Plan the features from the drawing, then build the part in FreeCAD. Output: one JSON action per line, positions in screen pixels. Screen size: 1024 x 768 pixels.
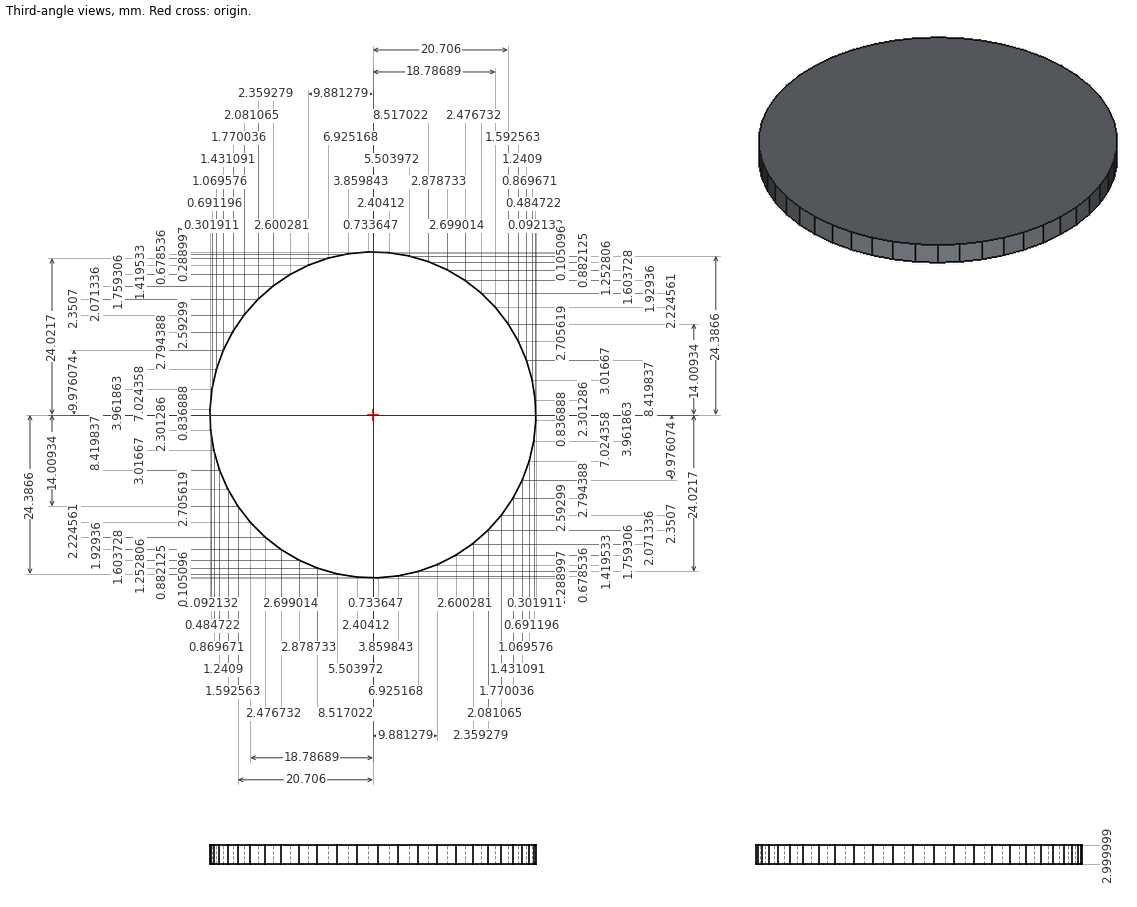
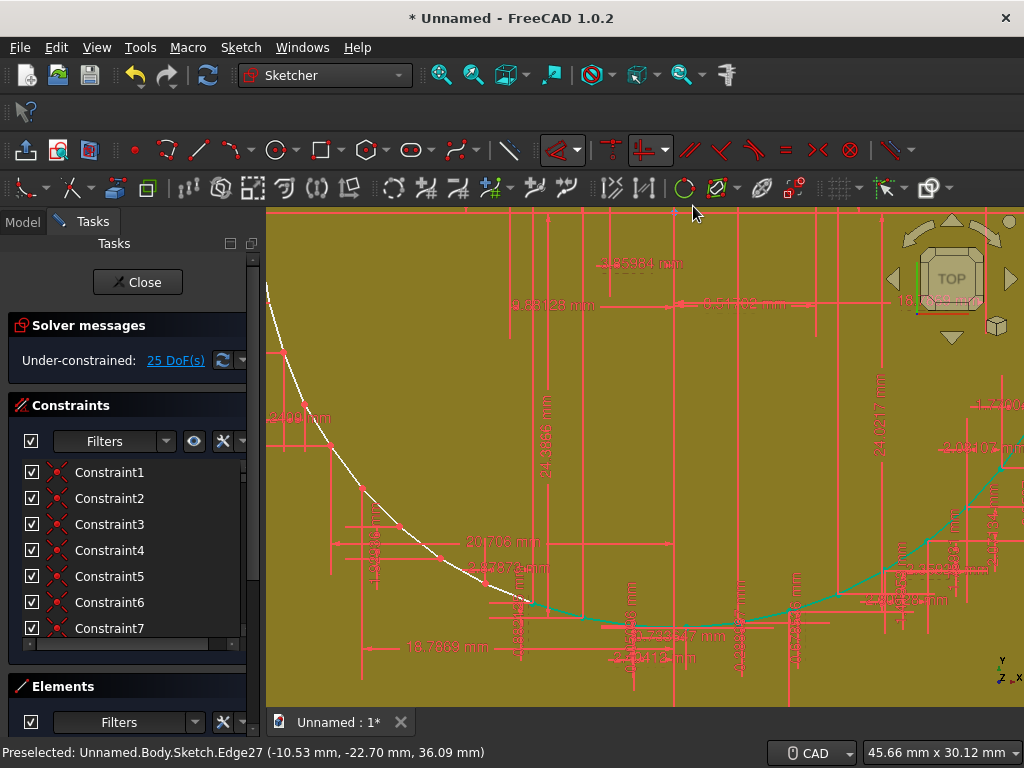
{"action": "scroll", "coordinate": [519, 597], "scroll_direction": "up", "scroll_amount": 4}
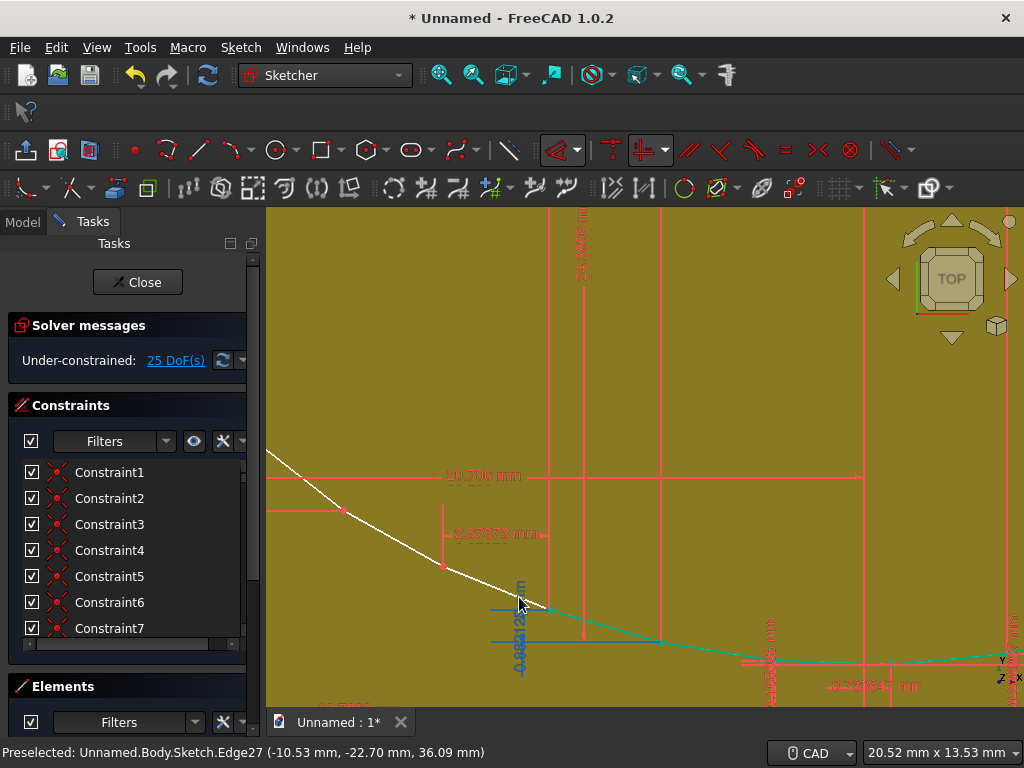
{"action": "left_click", "coordinate": [475, 579]}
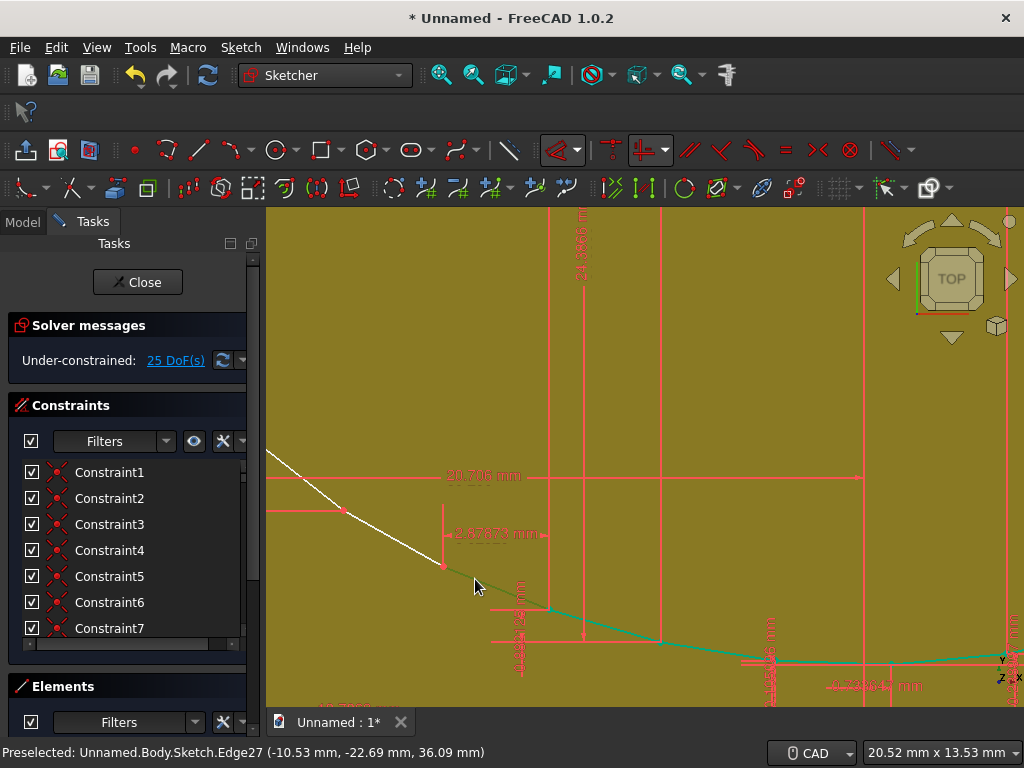
{"action": "left_click", "coordinate": [580, 150]}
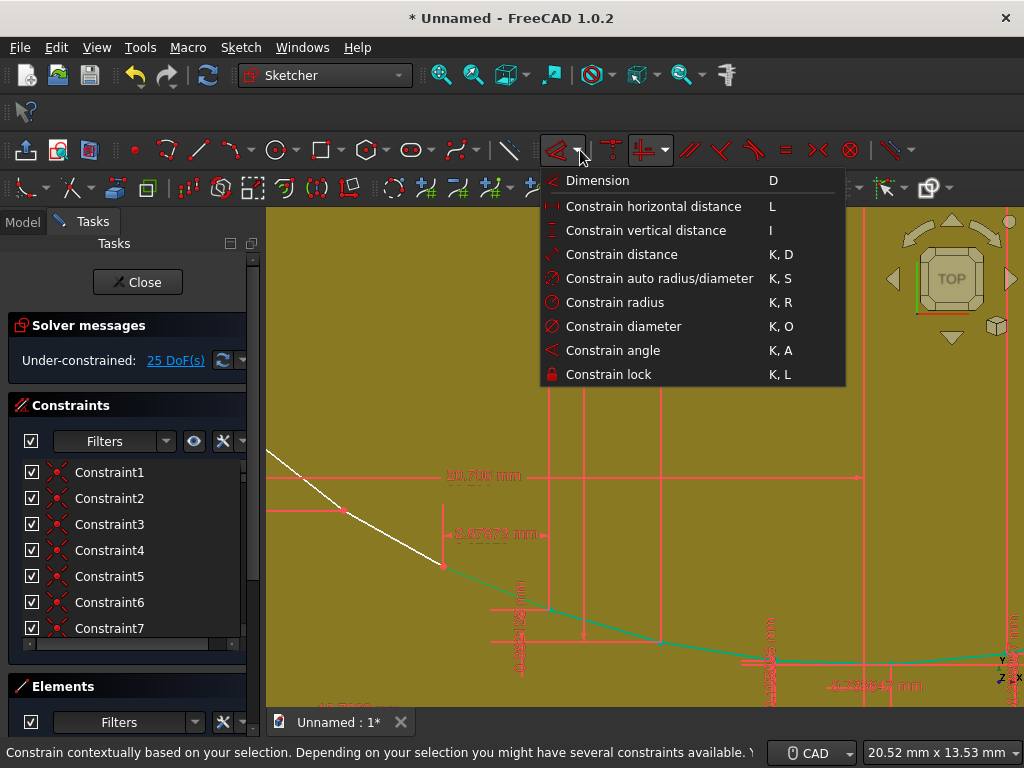
{"action": "left_click", "coordinate": [693, 230]}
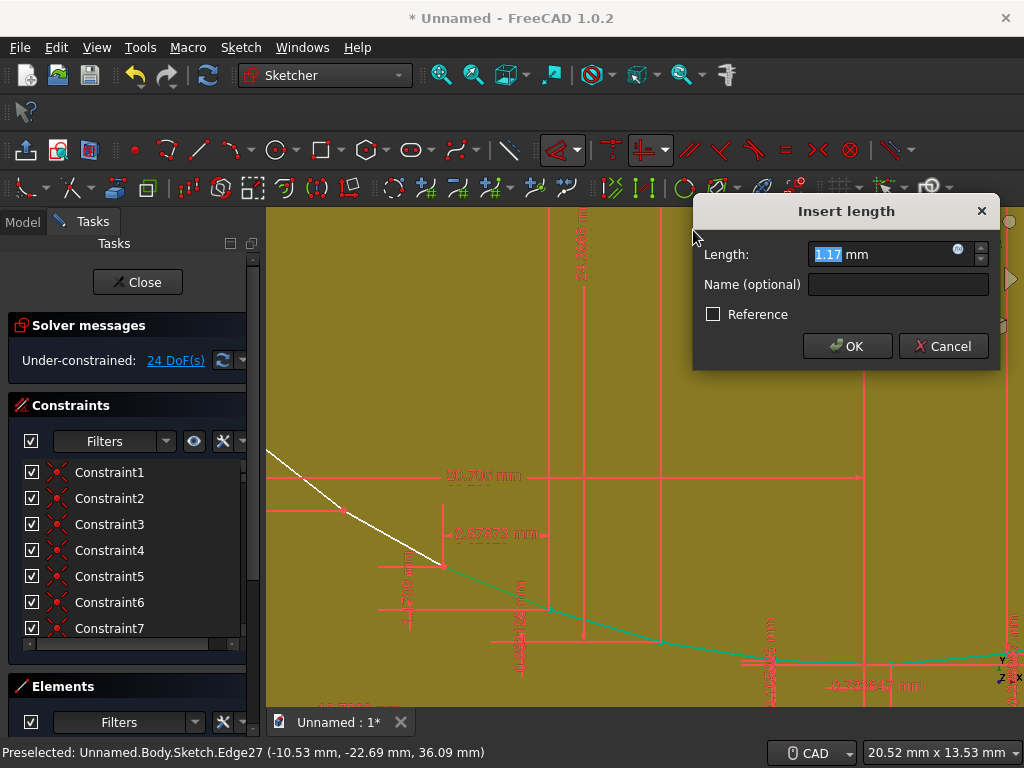
{"action": "type", "text": "1.252806"}
{"action": "key", "text": "Return"}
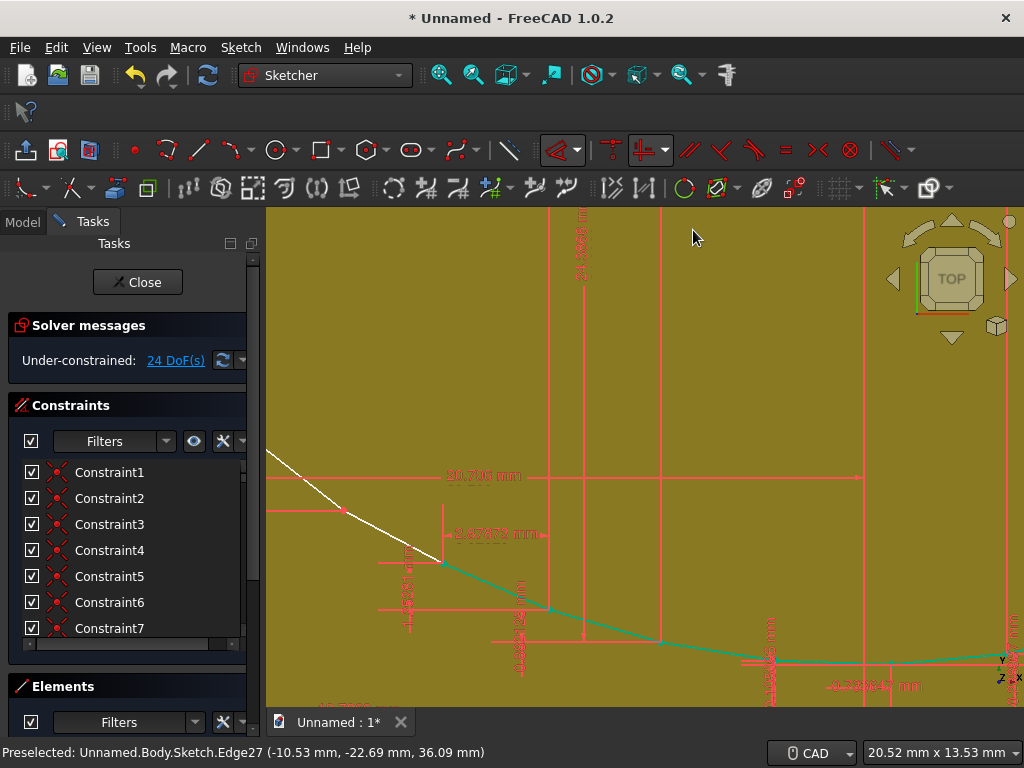
{"action": "left_click", "coordinate": [374, 527]}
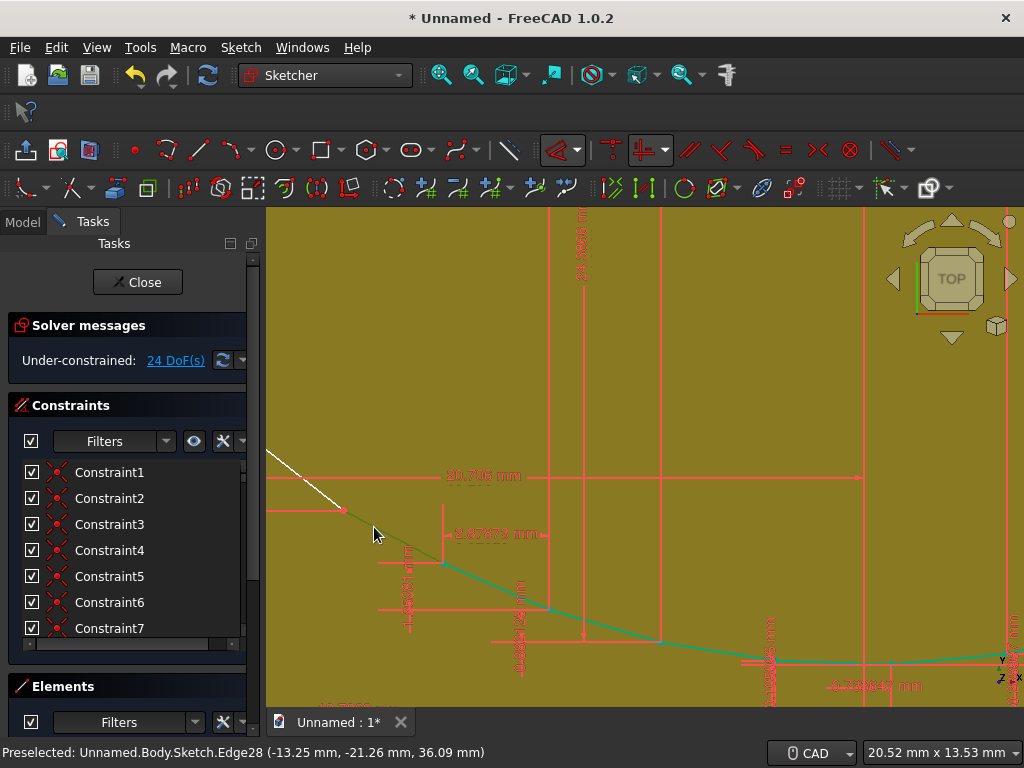
{"action": "left_click", "coordinate": [580, 150]}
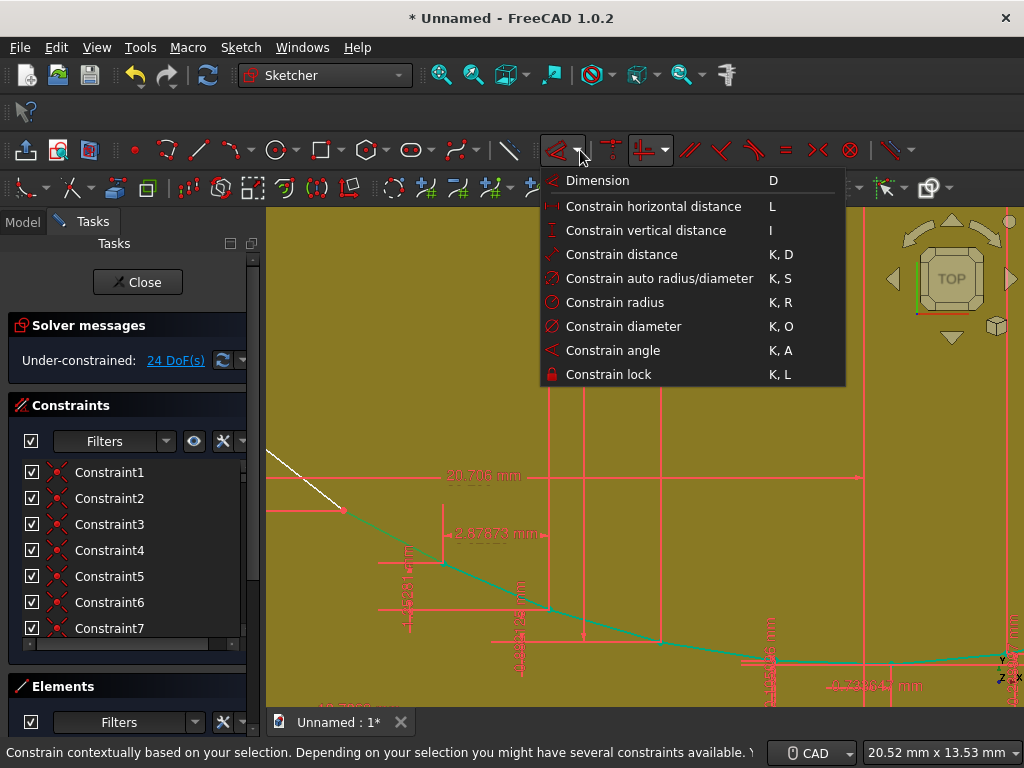
{"action": "left_click", "coordinate": [693, 206]}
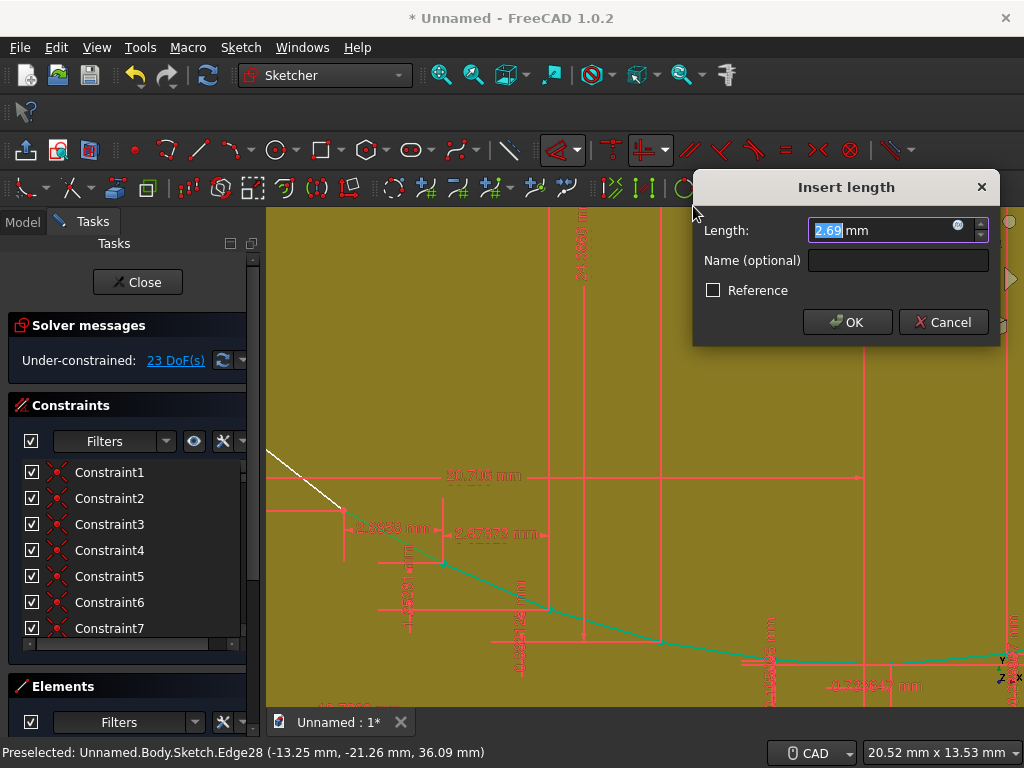
{"action": "type", "text": "2.699014"}
{"action": "key", "text": "Return"}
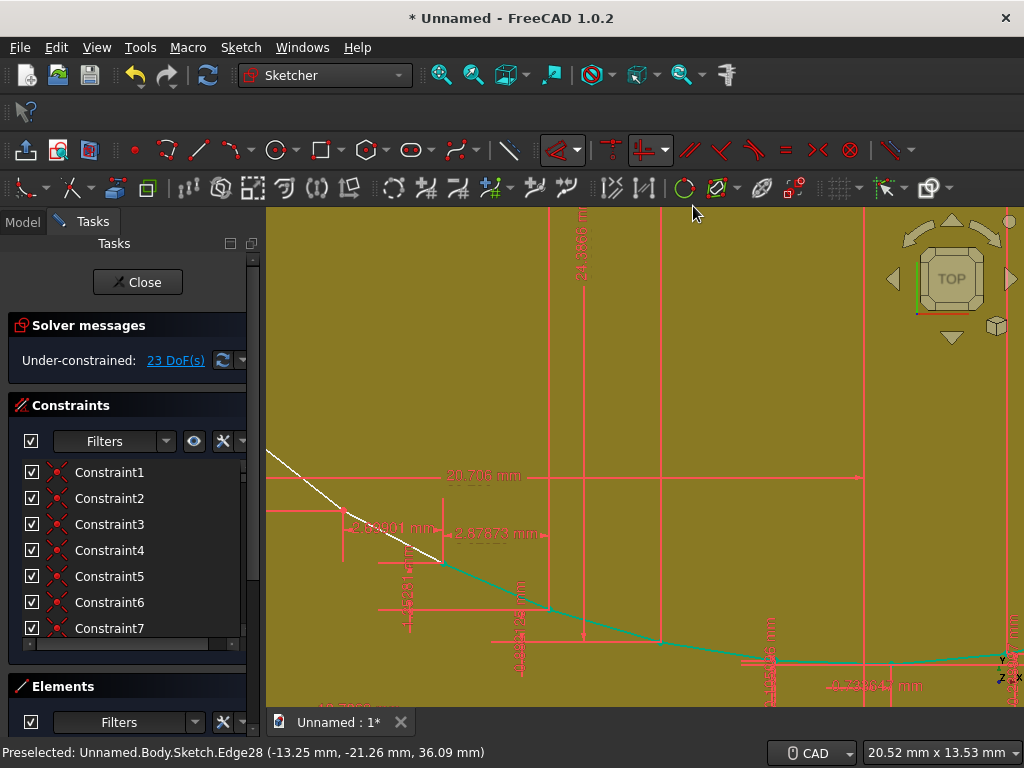
{"action": "left_click", "coordinate": [403, 542]}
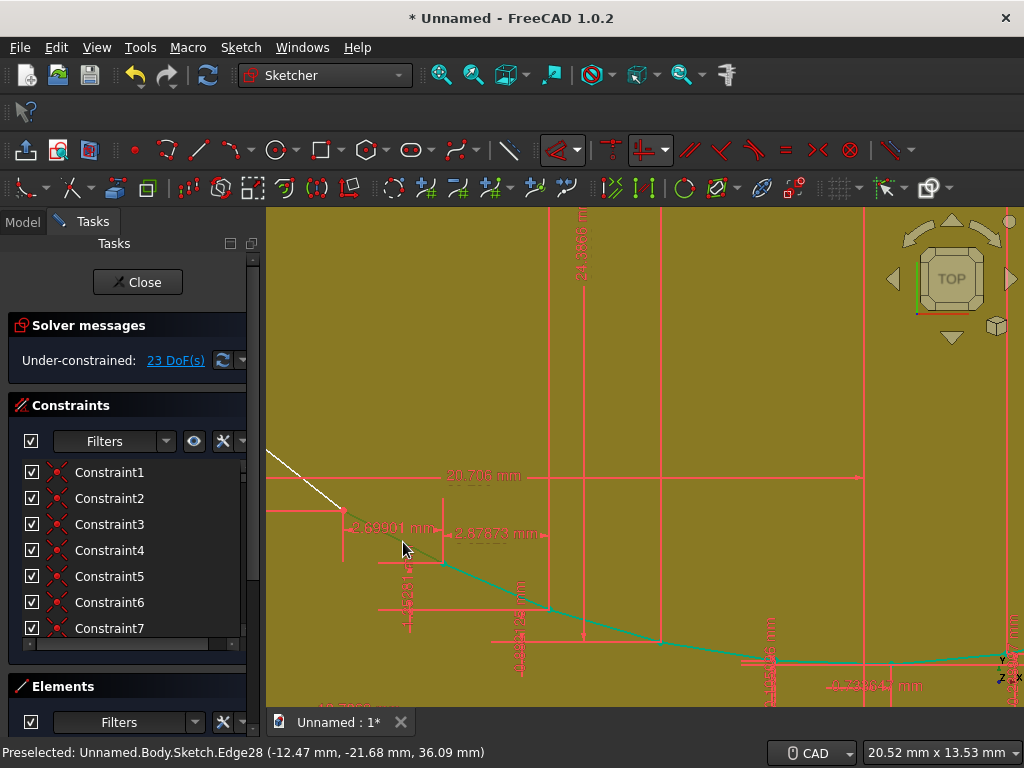
{"action": "key", "text": "i"}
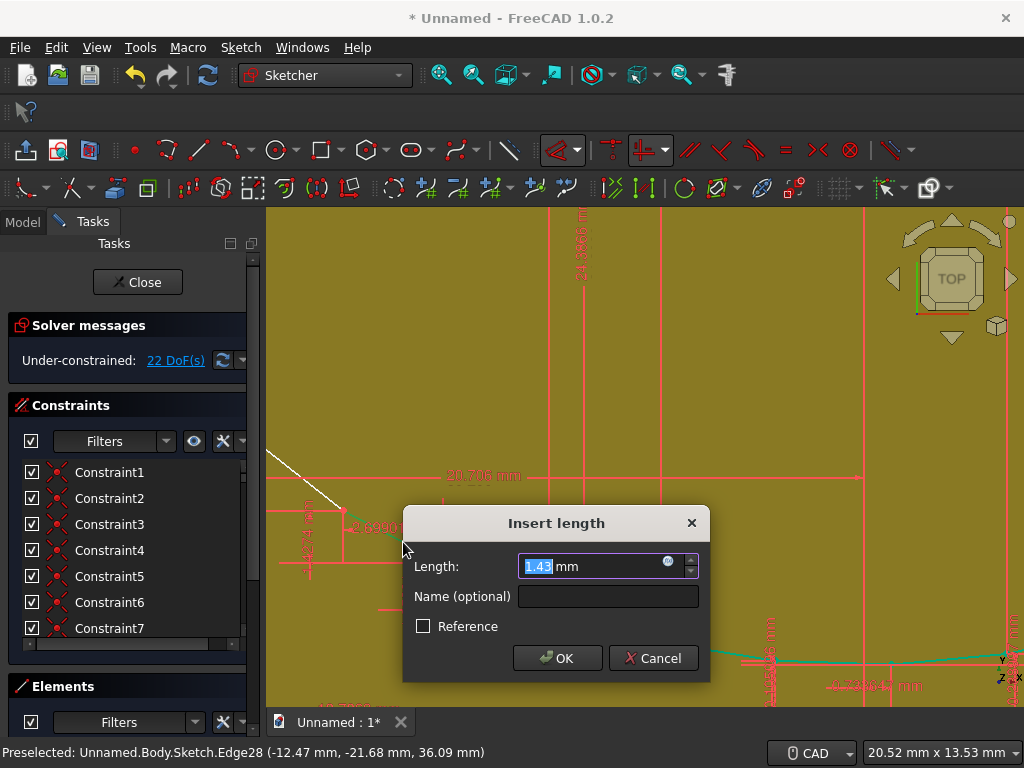
{"action": "type", "text": "1.603728"}
{"action": "key", "text": "Return"}